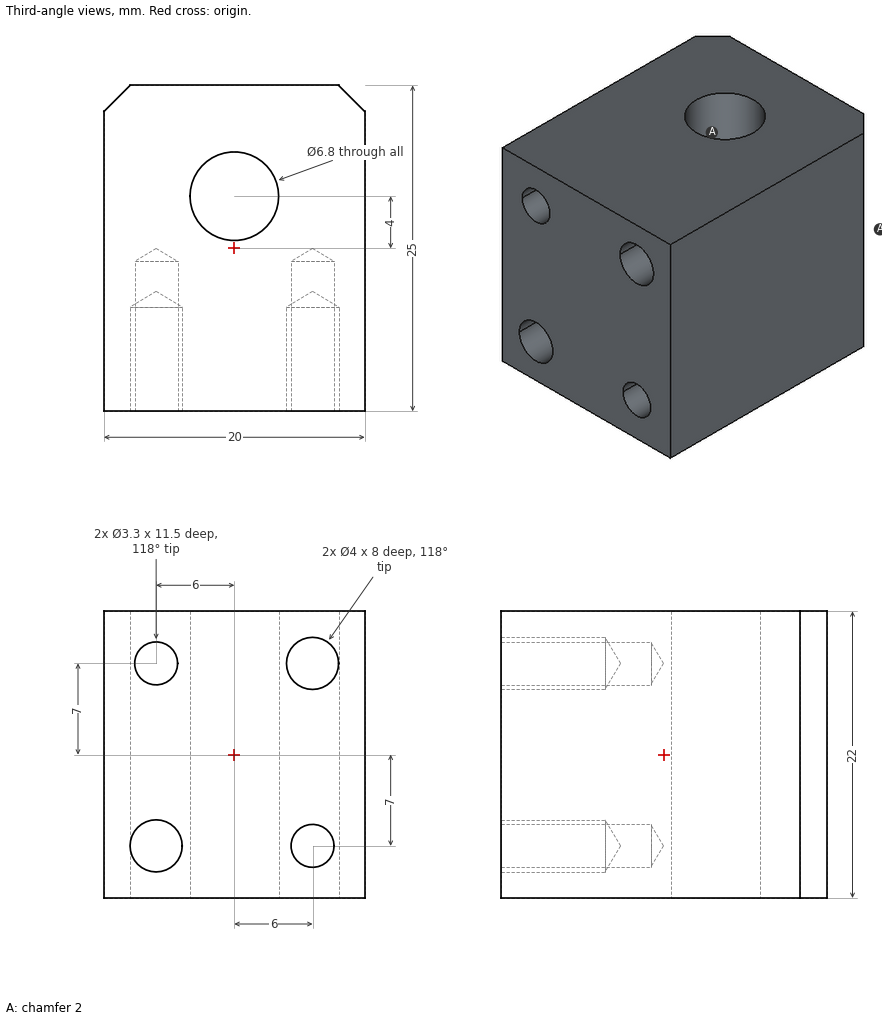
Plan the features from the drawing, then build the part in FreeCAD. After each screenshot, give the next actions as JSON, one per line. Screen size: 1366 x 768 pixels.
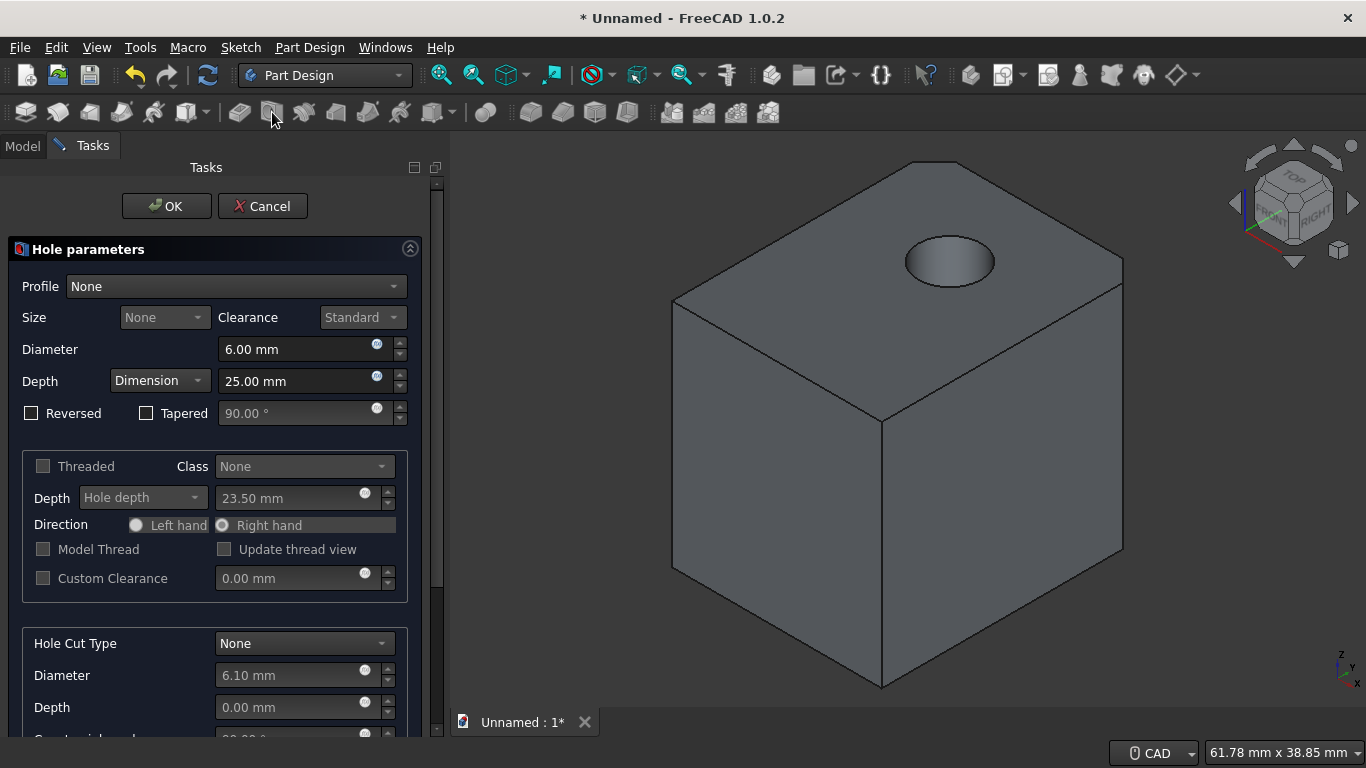
{"action": "triple_click", "coordinate": [305, 349]}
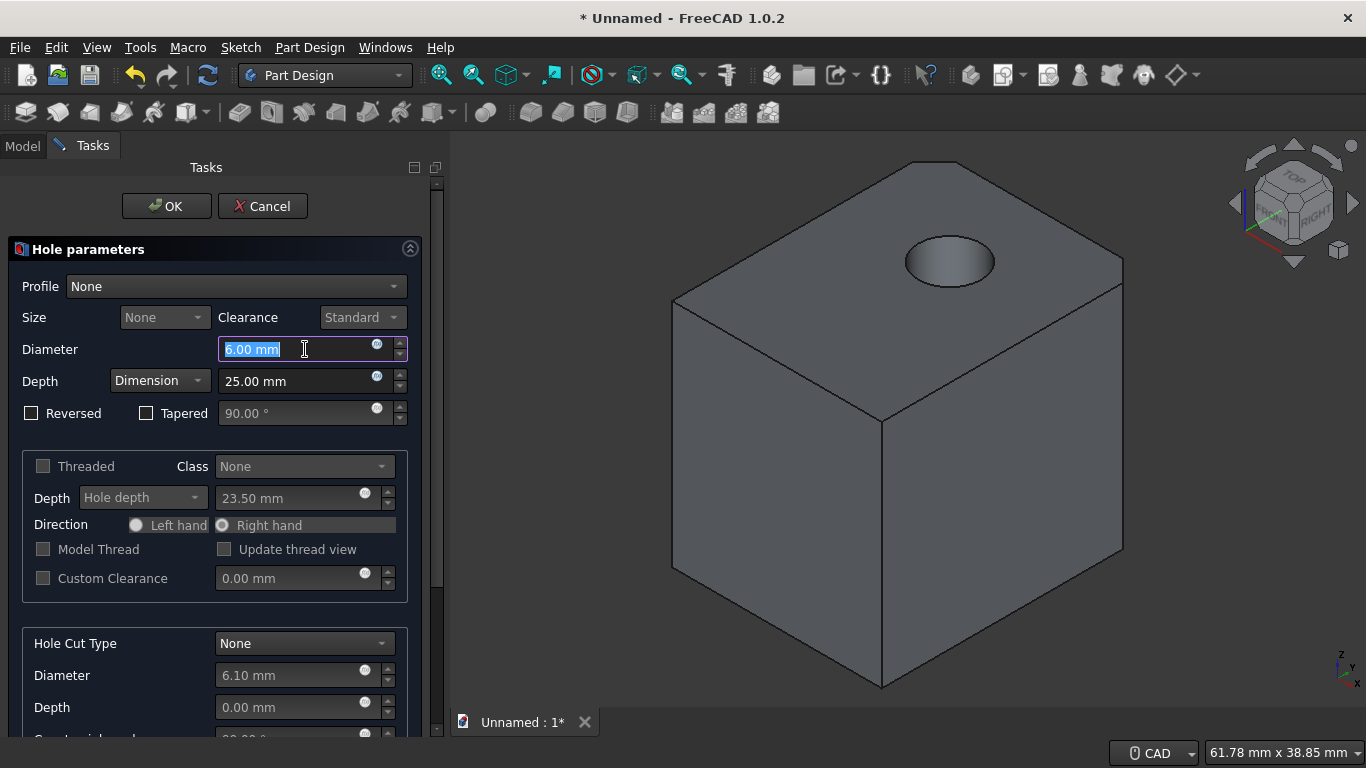
{"action": "type", "text": "6.8"}
{"action": "key", "text": "Tab"}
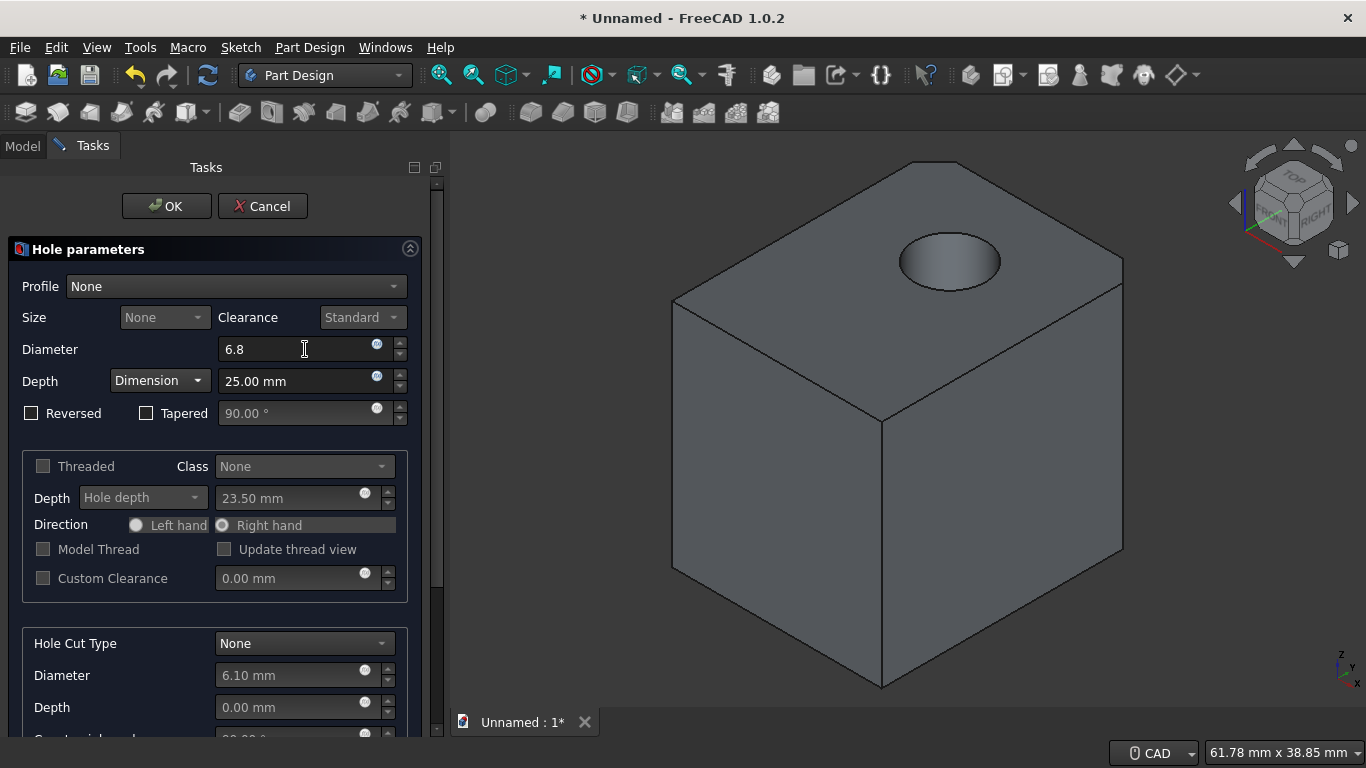
{"action": "left_click", "coordinate": [161, 380]}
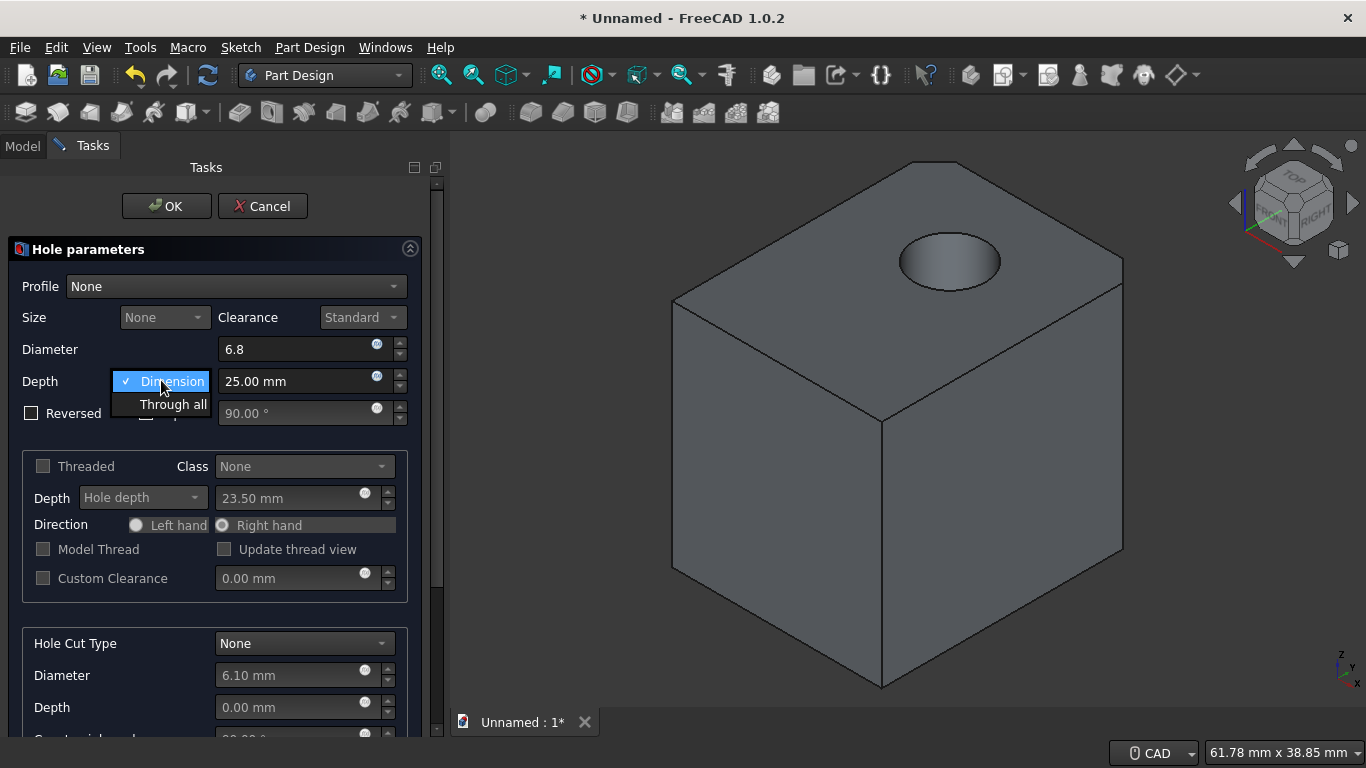
{"action": "left_click", "coordinate": [160, 404]}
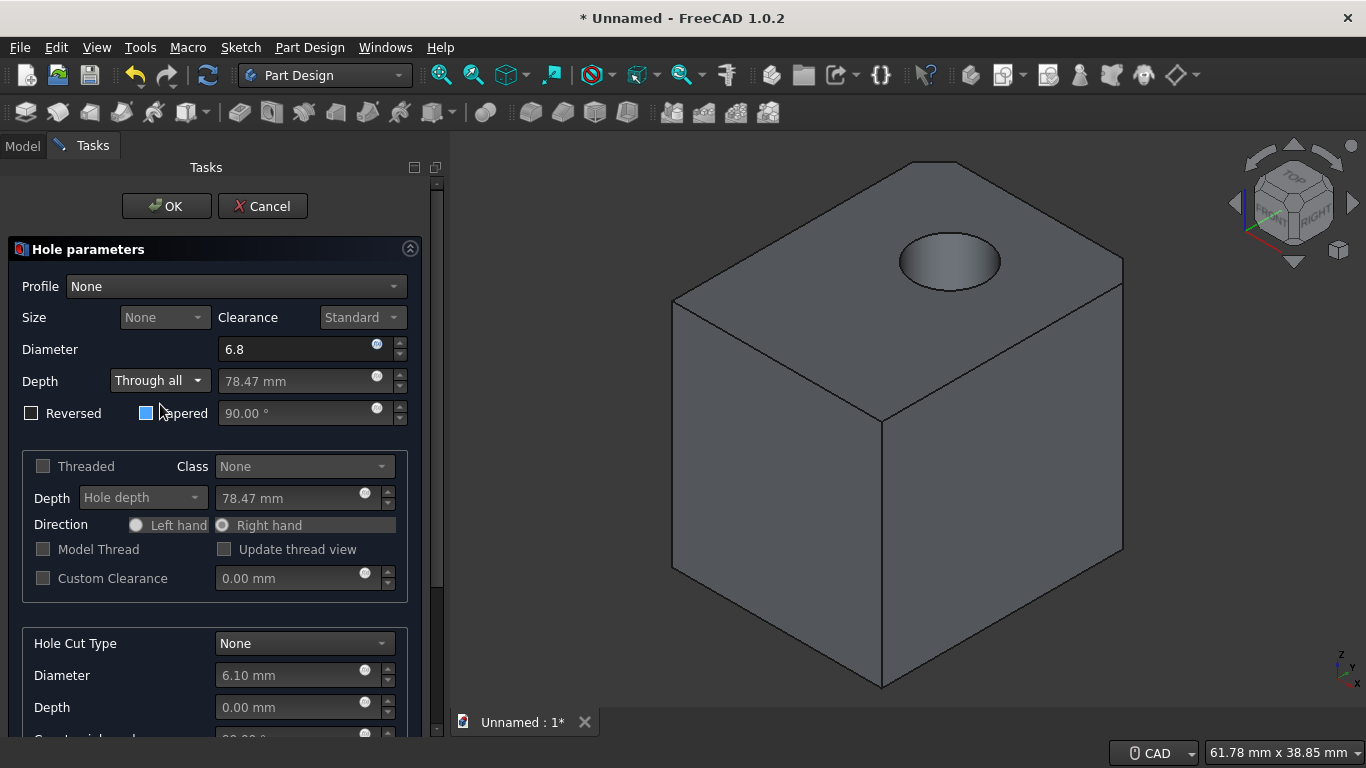
{"action": "left_click", "coordinate": [167, 206]}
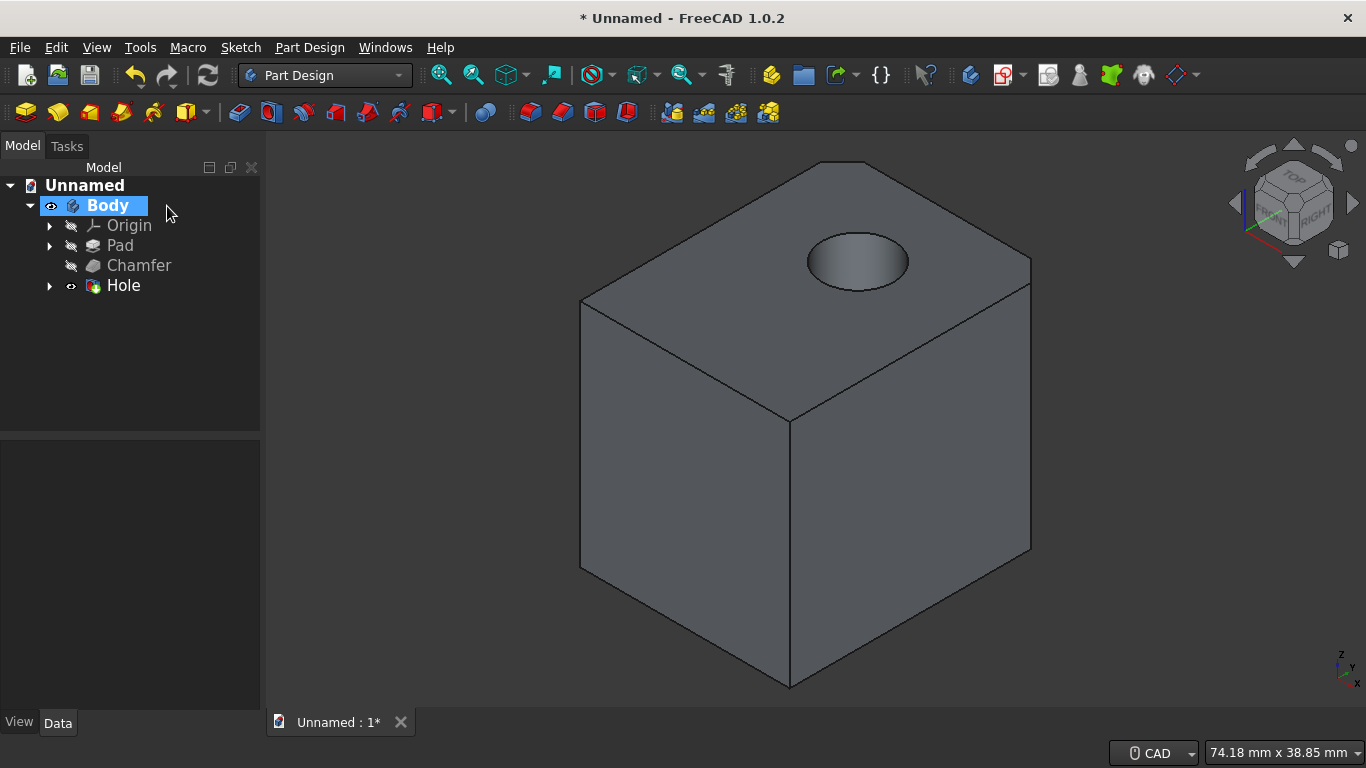
{"action": "left_click", "coordinate": [685, 494]}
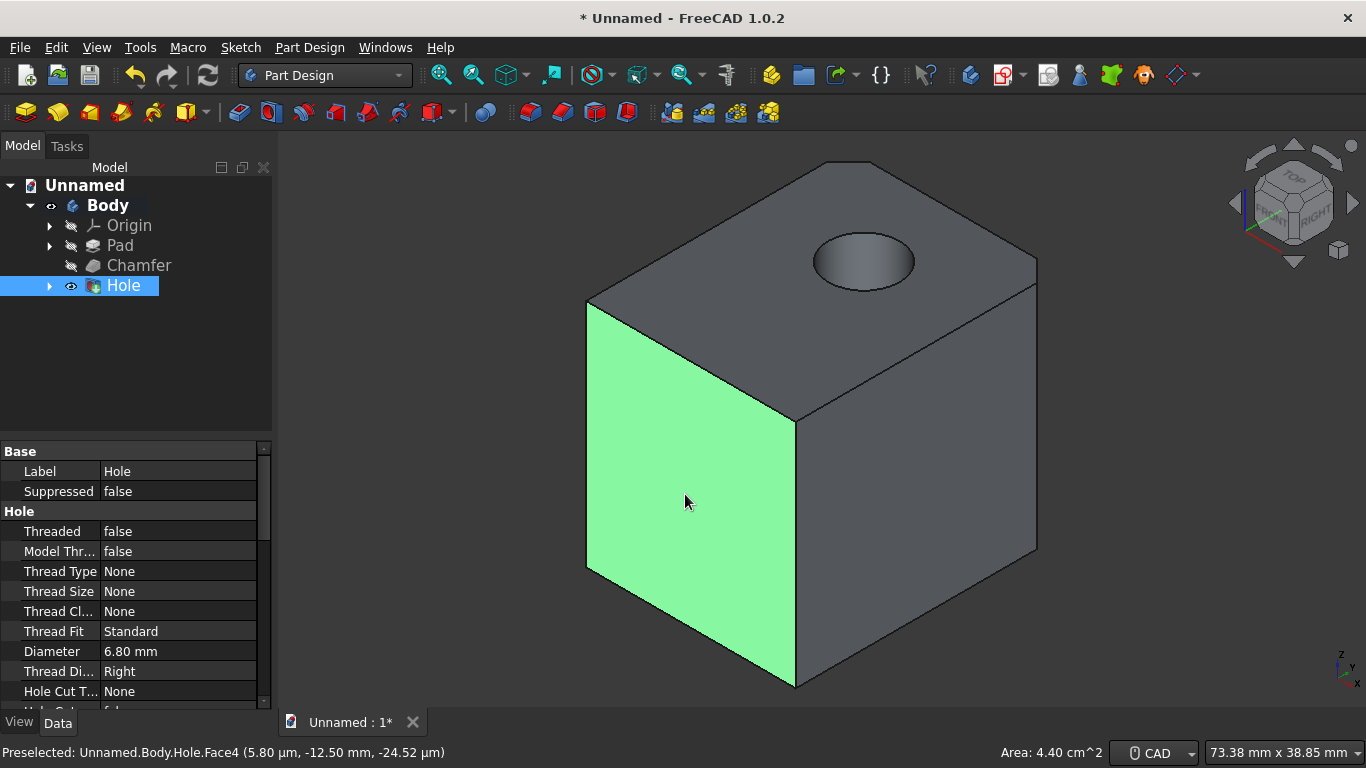
{"action": "left_click", "coordinate": [1004, 76]}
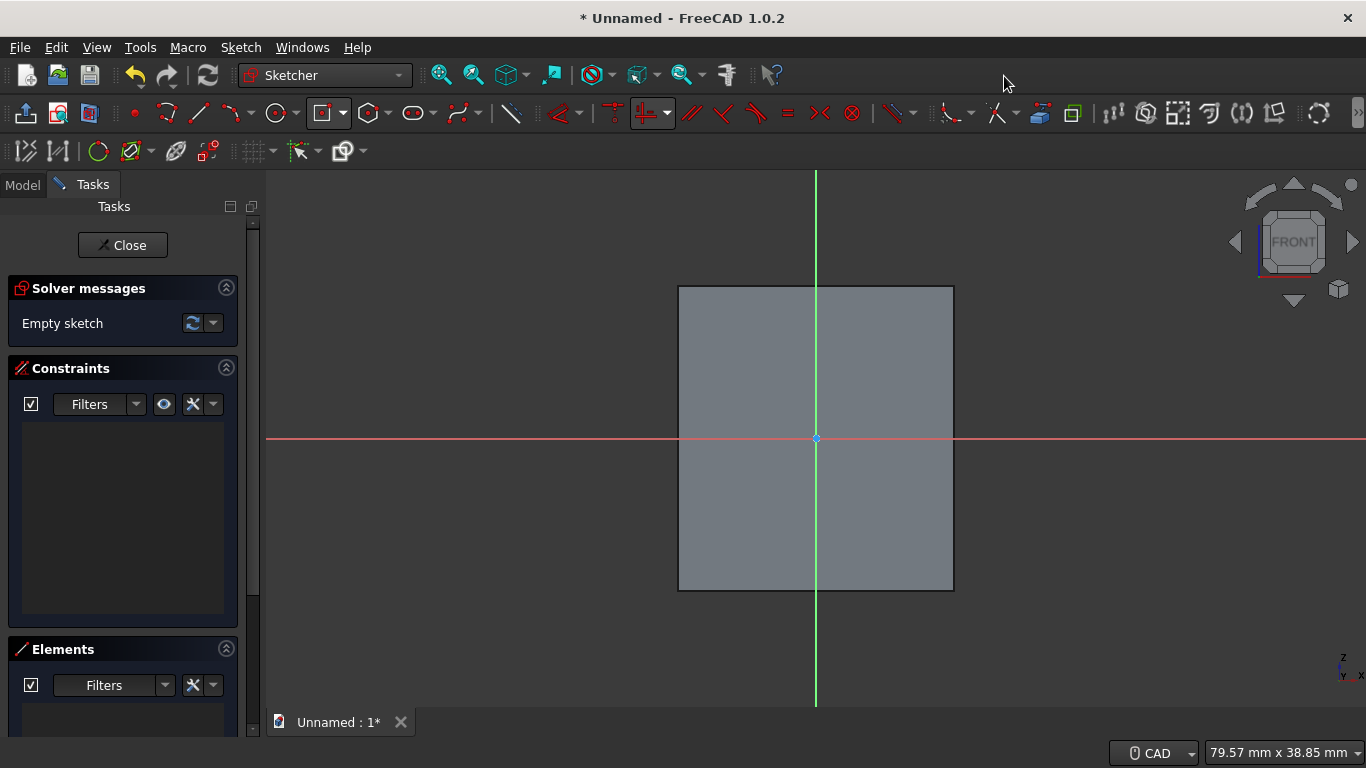
{"action": "scroll", "coordinate": [955, 438], "scroll_direction": "up", "scroll_amount": 2}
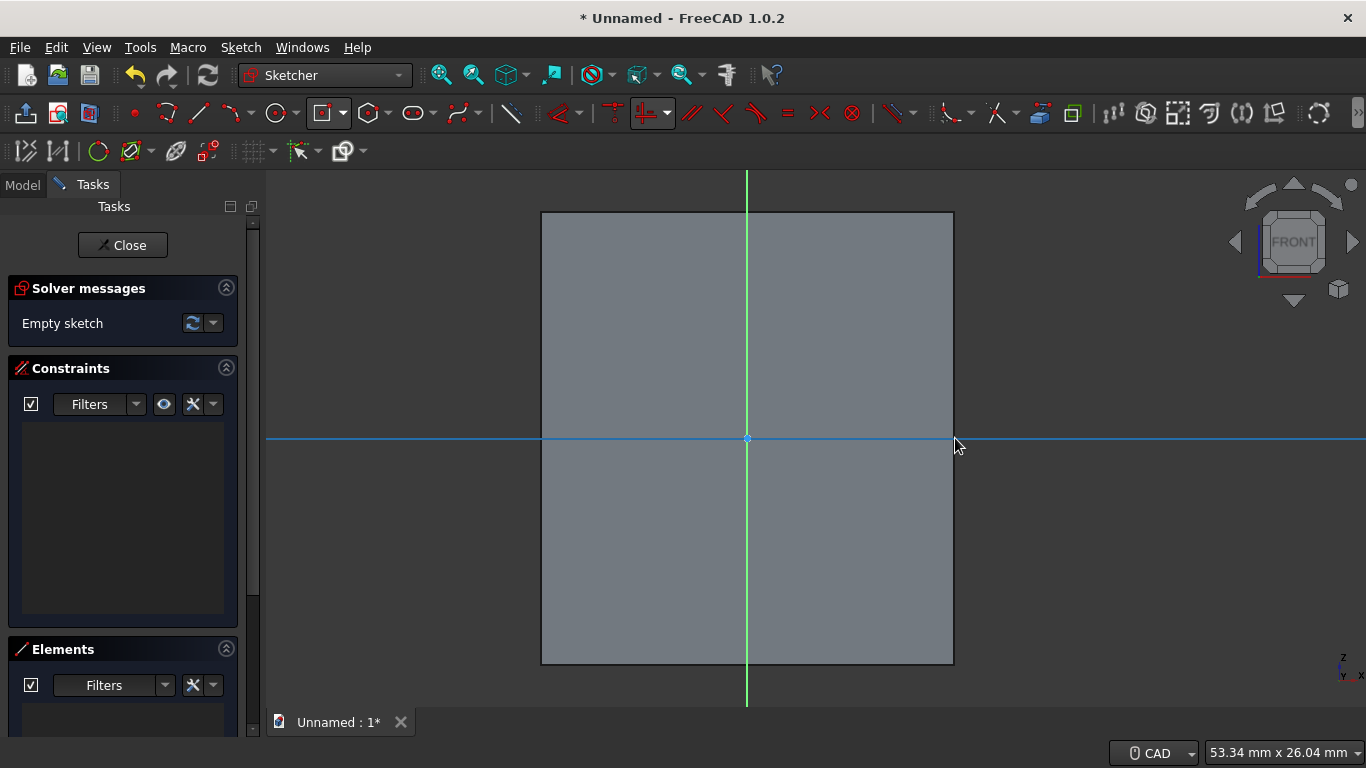
{"action": "left_click", "coordinate": [276, 114]}